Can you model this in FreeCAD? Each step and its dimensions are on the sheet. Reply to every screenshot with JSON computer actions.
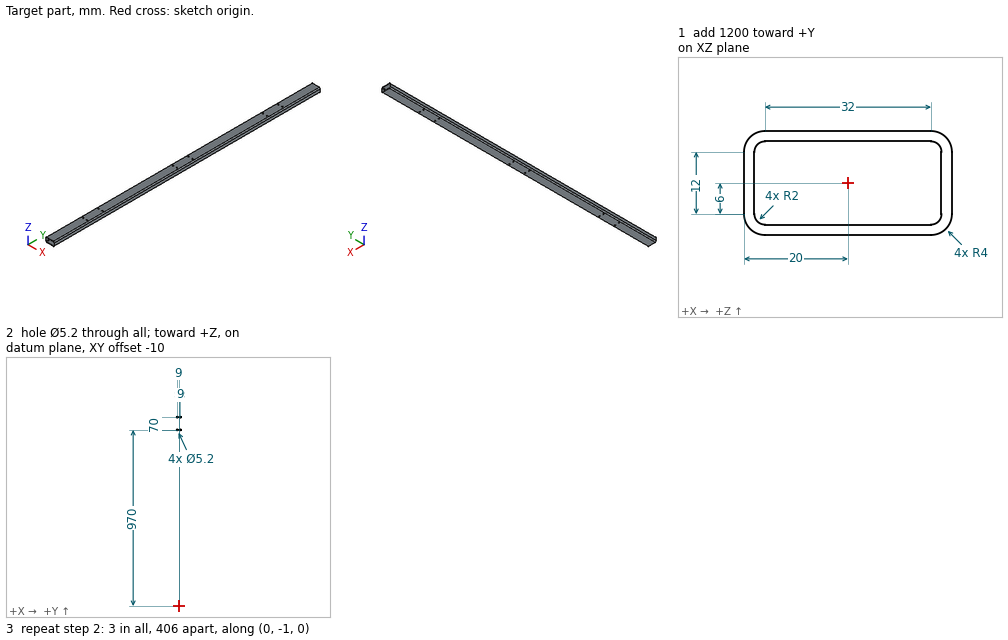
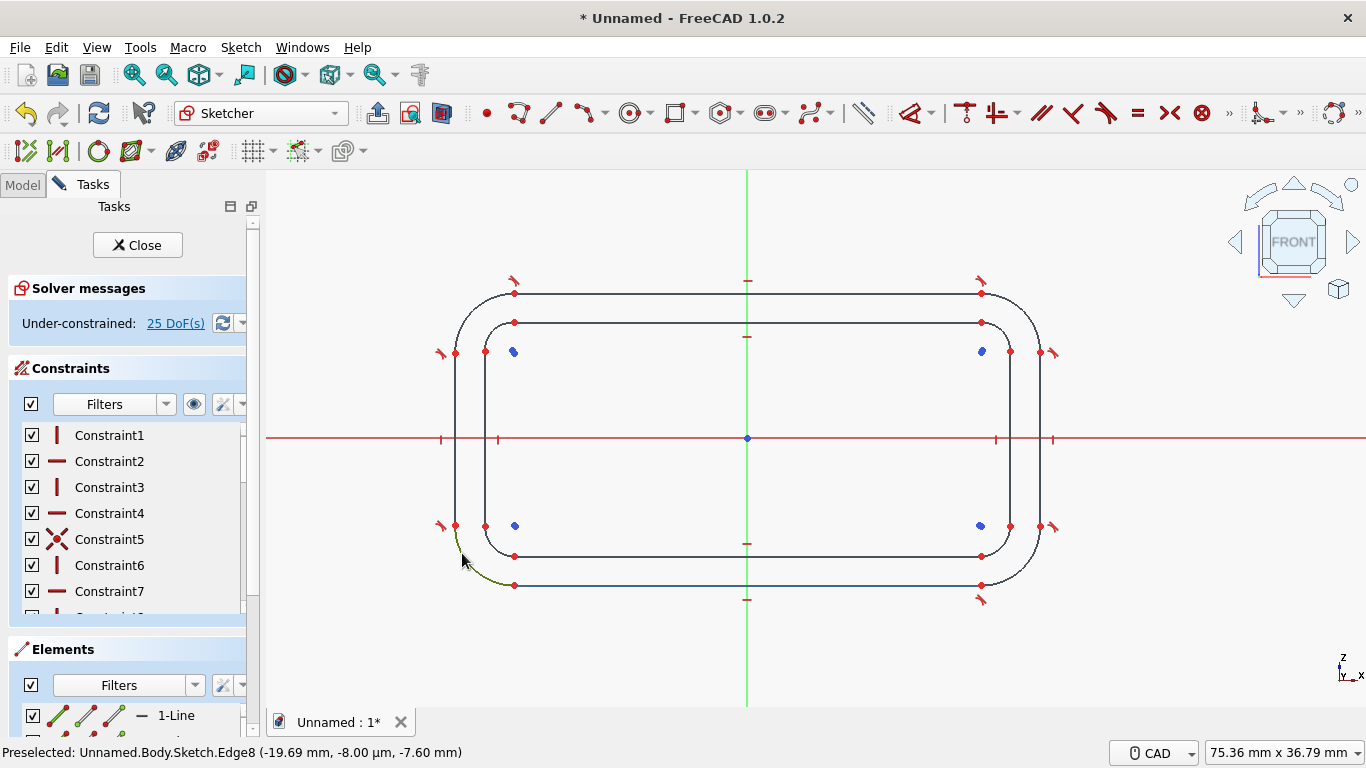
{"action": "left_click", "coordinate": [1106, 114]}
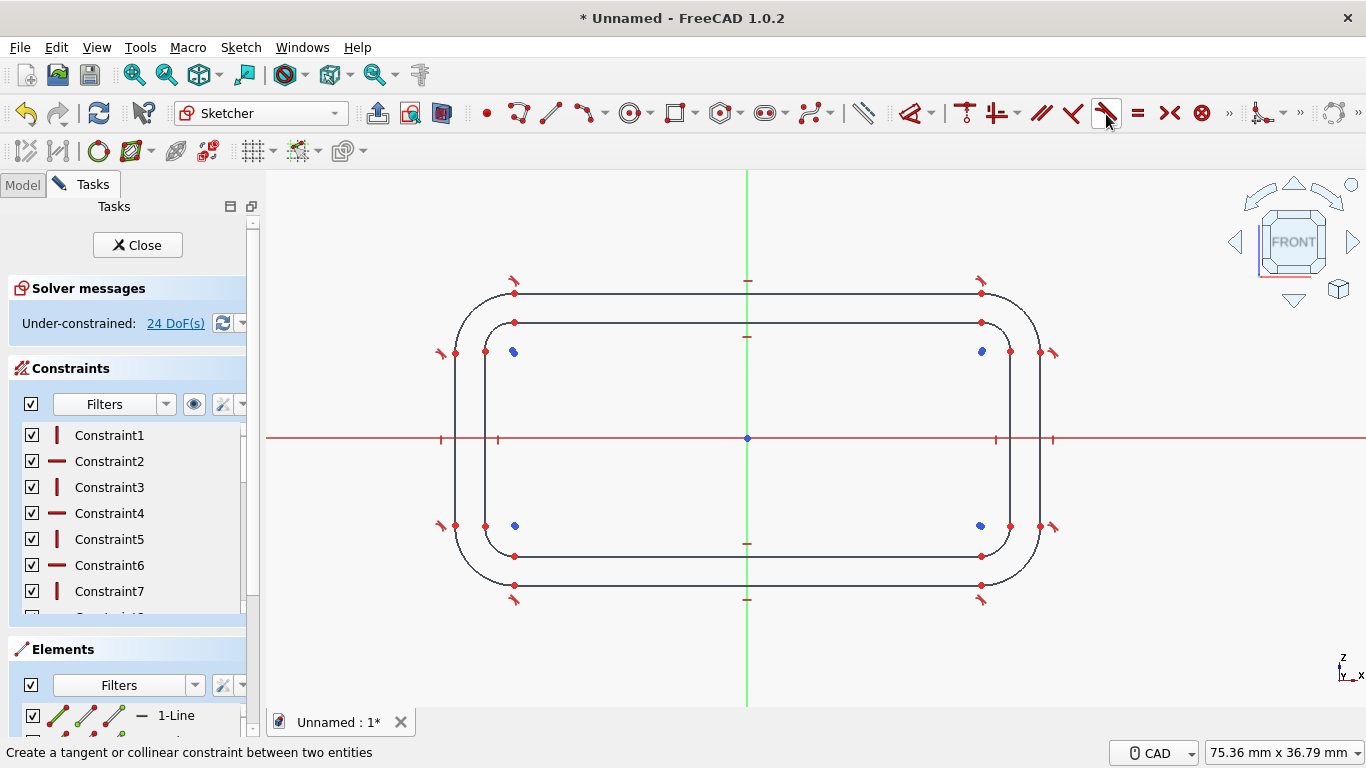
{"action": "left_click", "coordinate": [485, 404]}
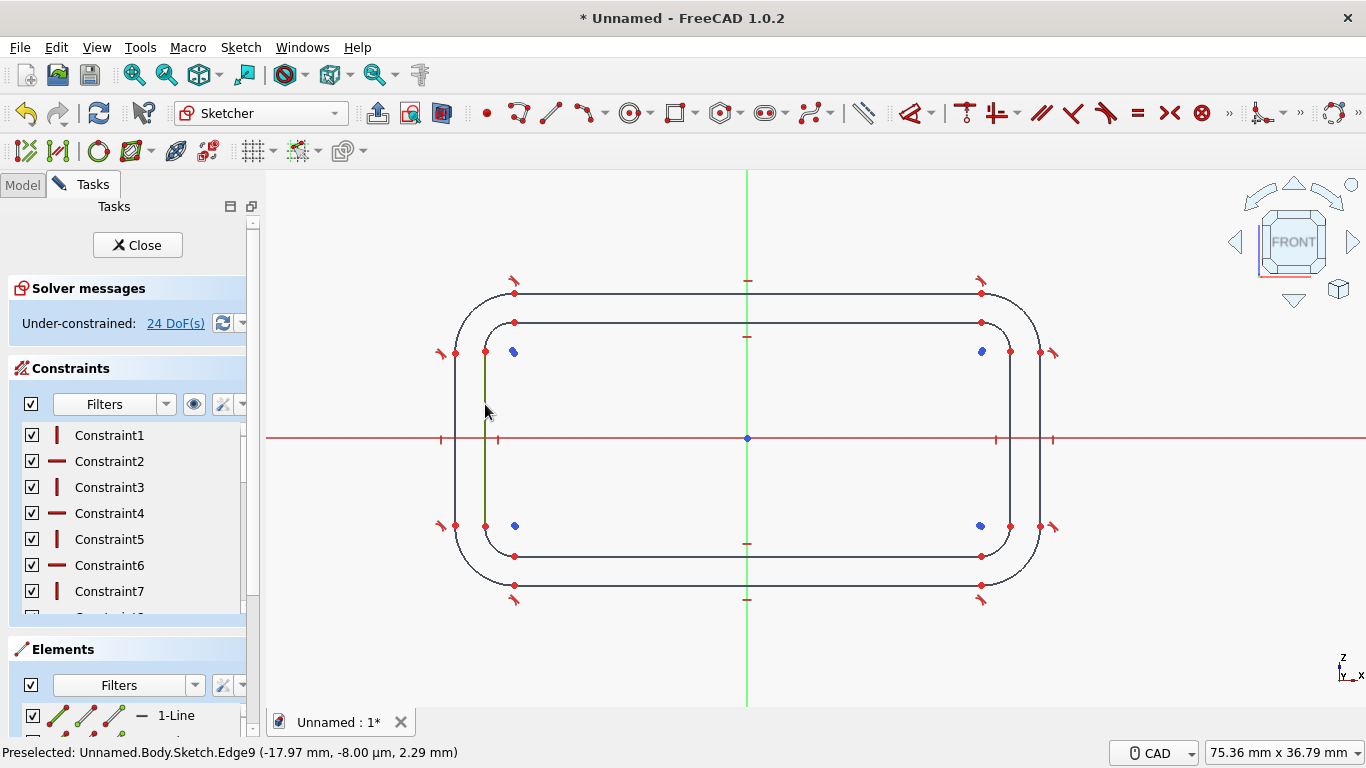
{"action": "left_click", "coordinate": [488, 540]}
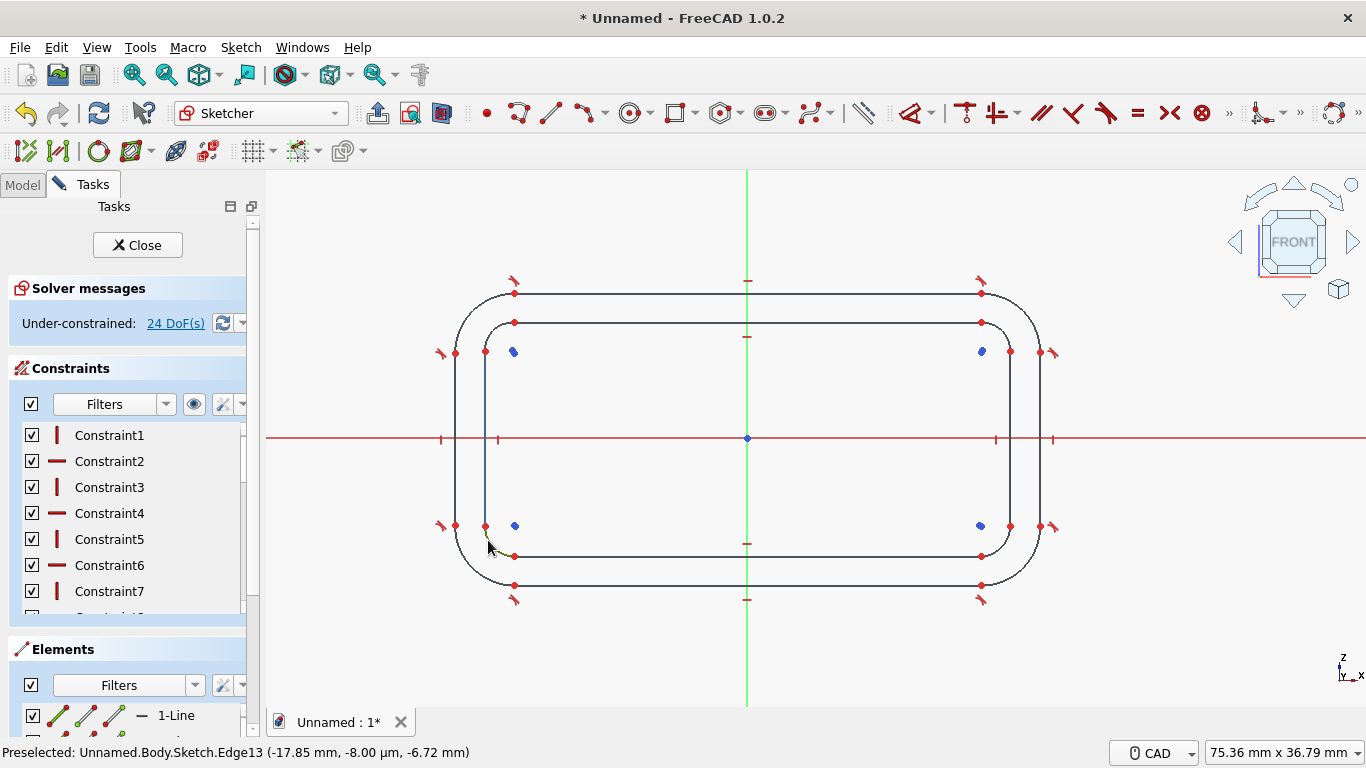
{"action": "left_click", "coordinate": [1106, 114]}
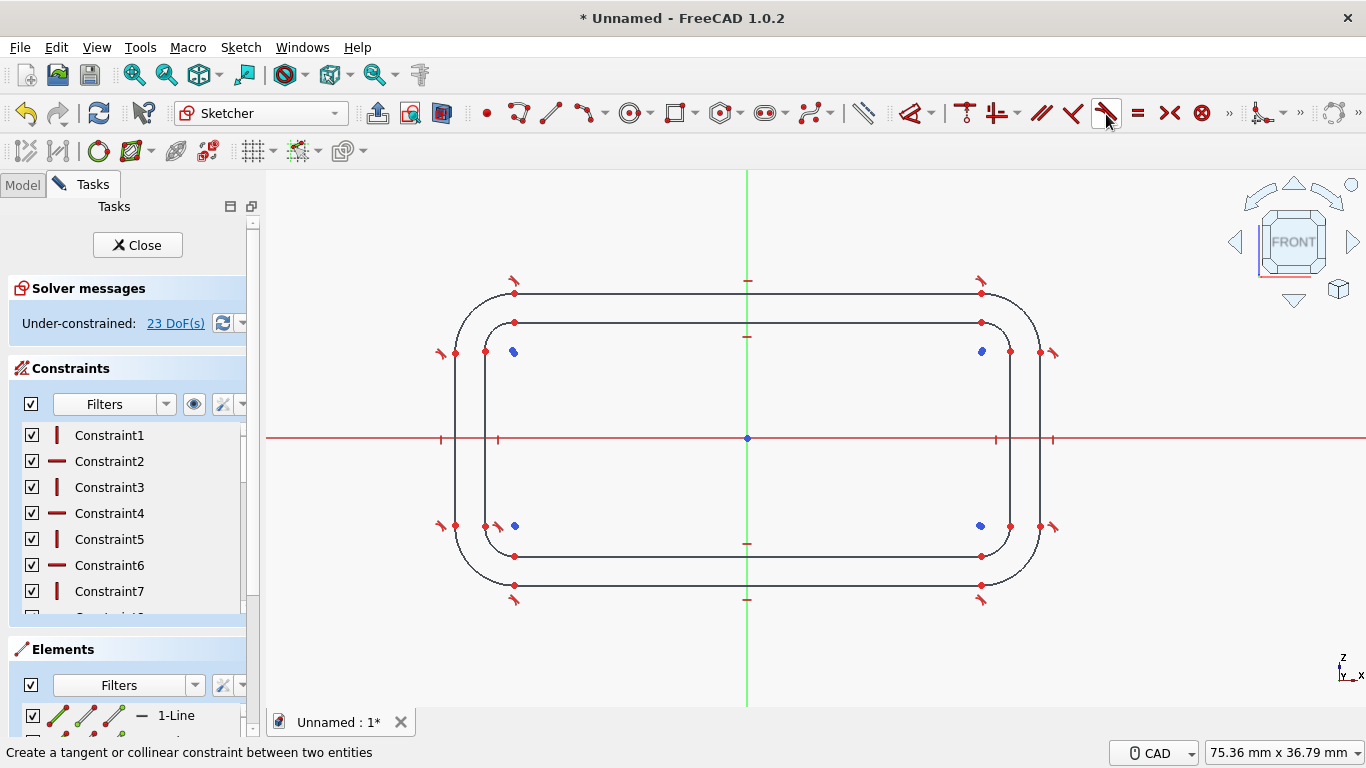
{"action": "left_click", "coordinate": [485, 404]}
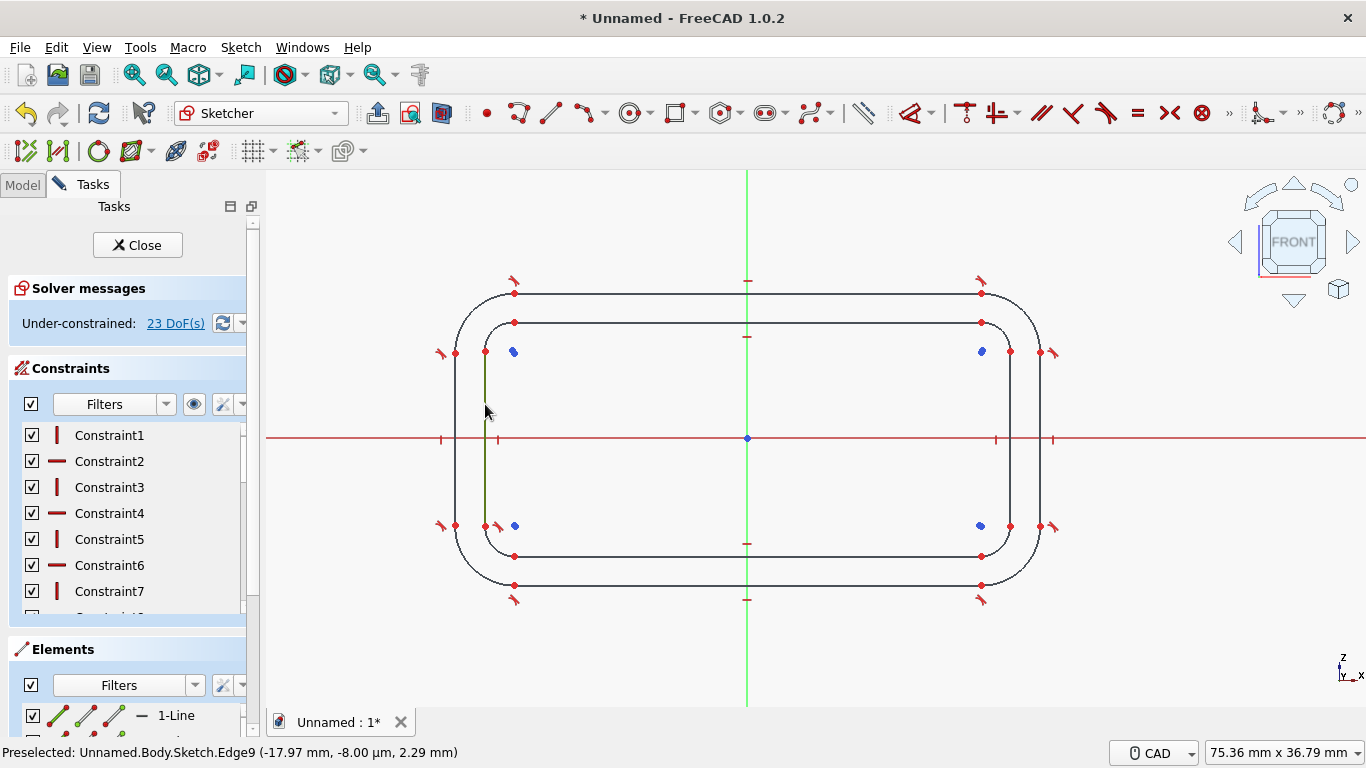
{"action": "left_click", "coordinate": [501, 325]}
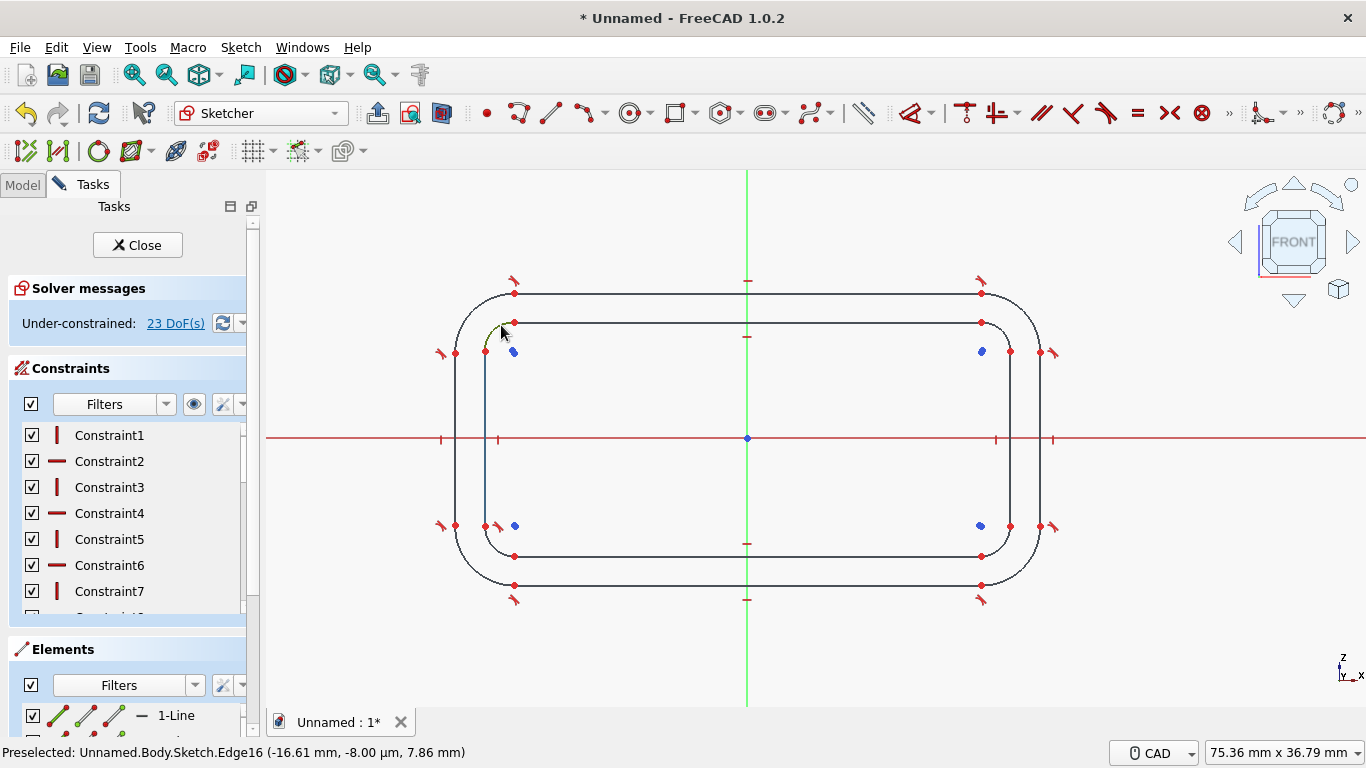
{"action": "key", "text": "t"}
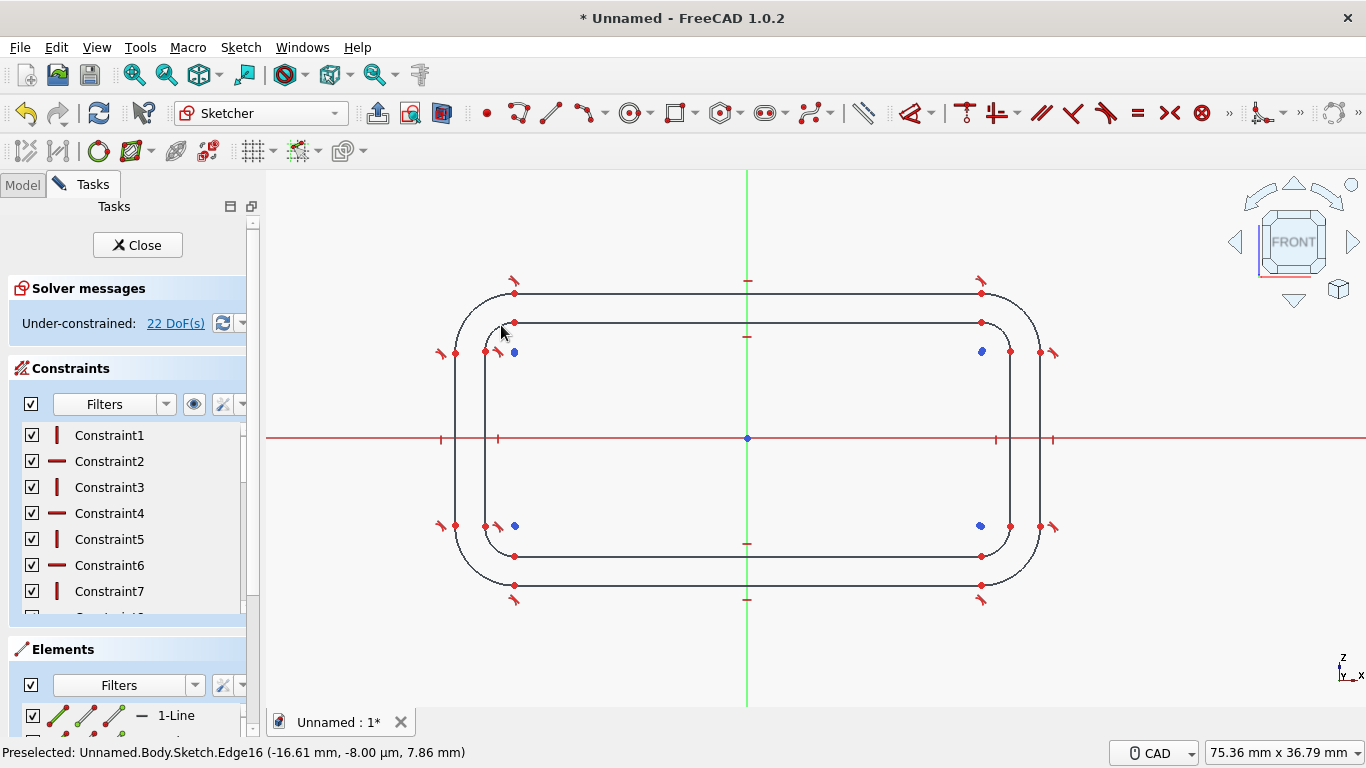
{"action": "left_click", "coordinate": [654, 557]}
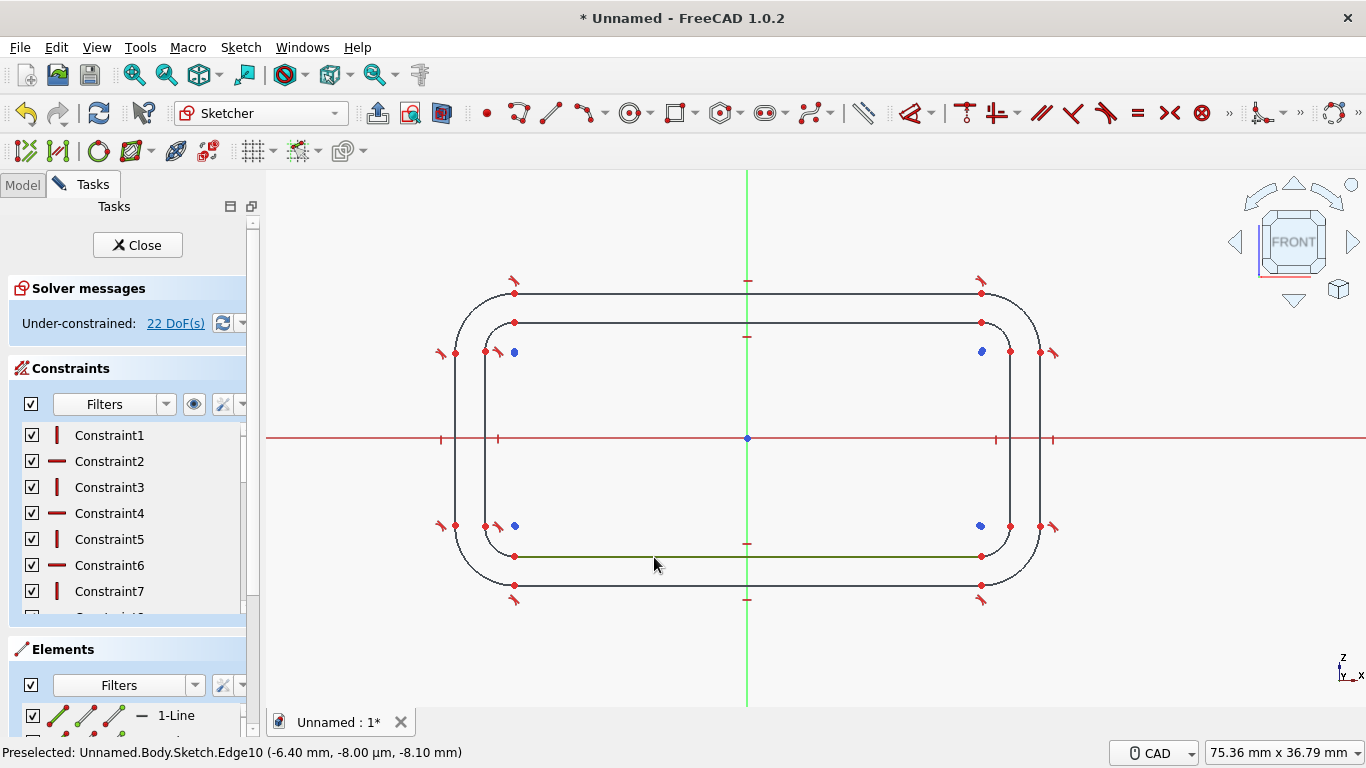
{"action": "left_click", "coordinate": [488, 540]}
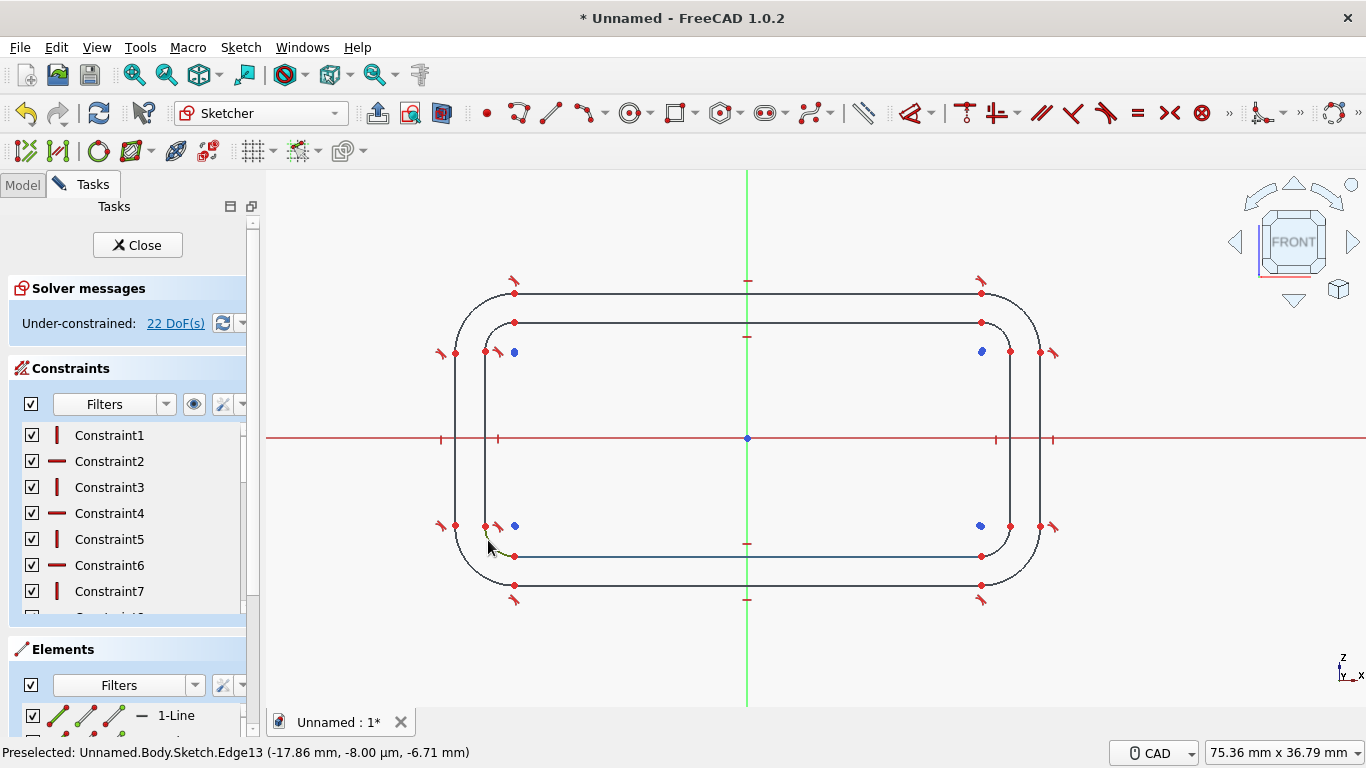
{"action": "left_click", "coordinate": [1106, 114]}